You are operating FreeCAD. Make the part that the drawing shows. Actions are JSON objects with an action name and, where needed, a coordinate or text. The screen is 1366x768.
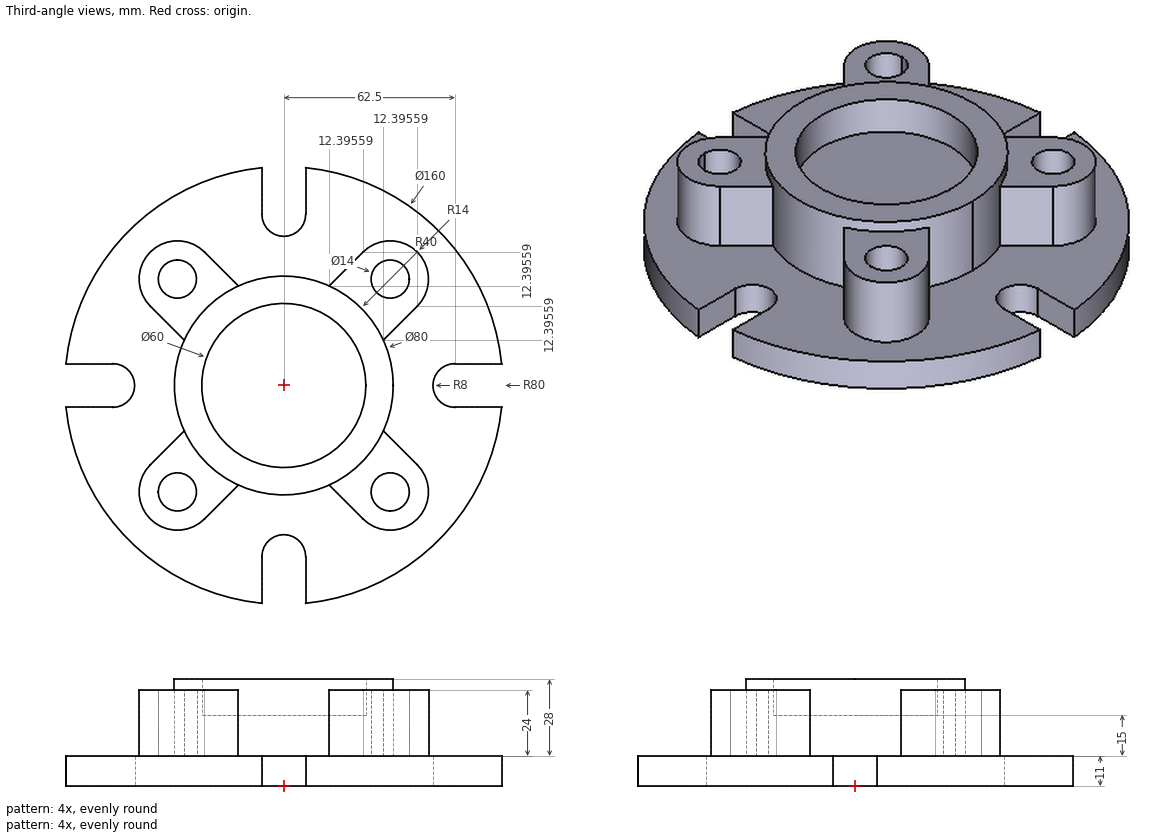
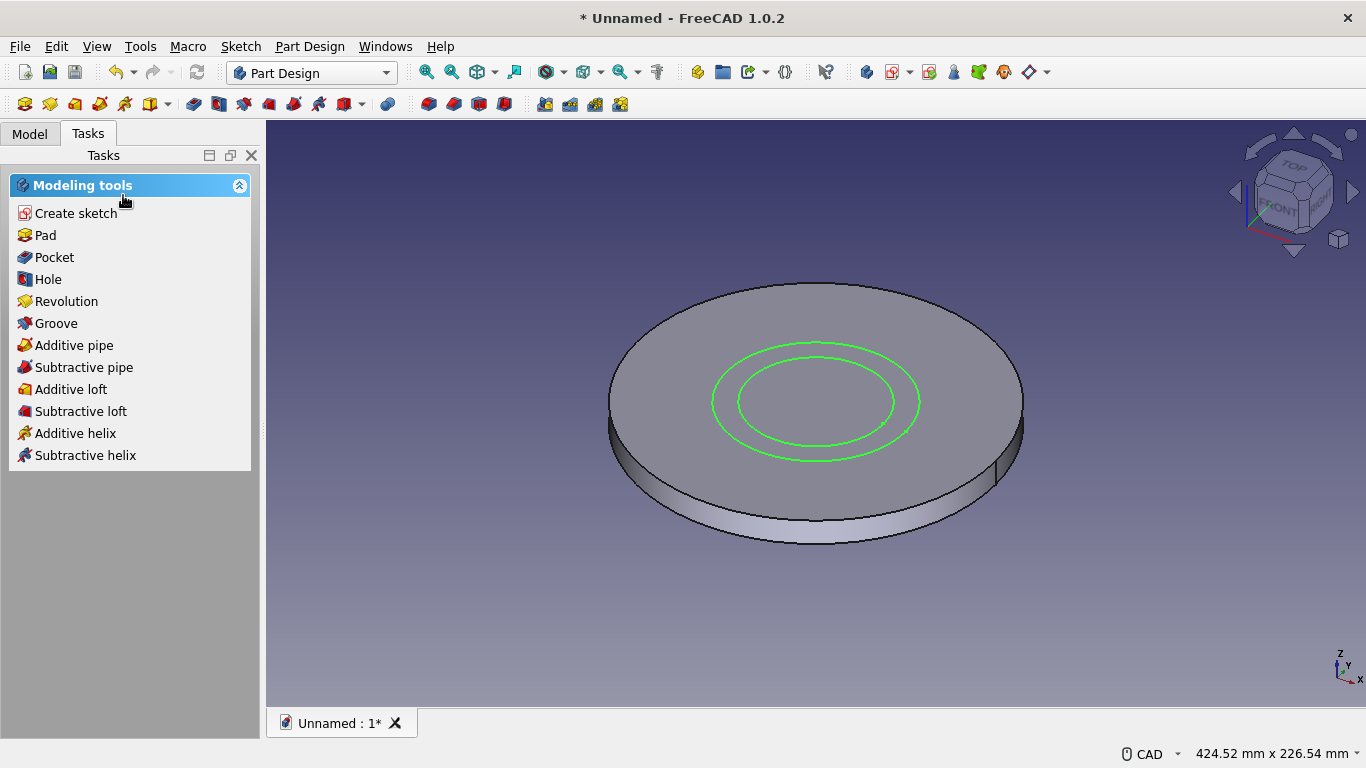
{"action": "left_click", "coordinate": [25, 104]}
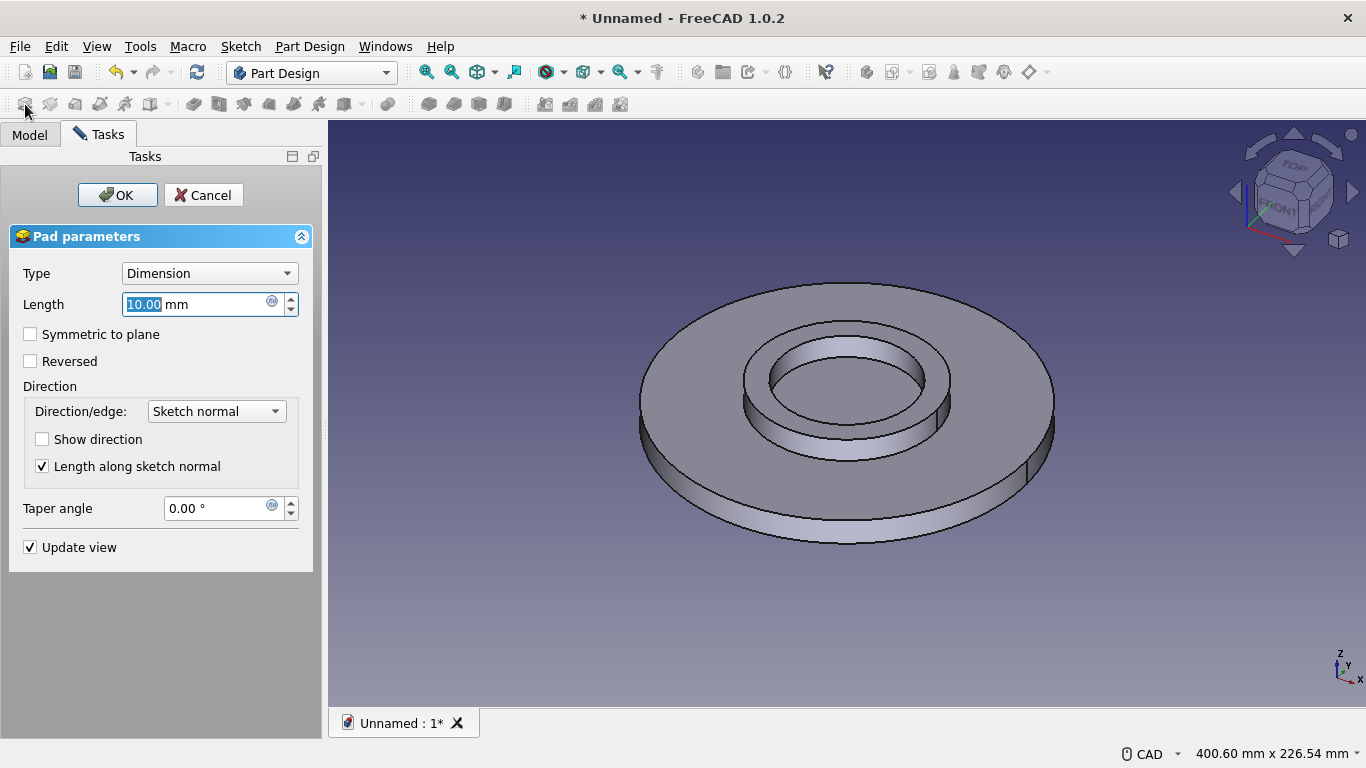
{"action": "type", "text": "28"}
{"action": "key", "text": "Tab"}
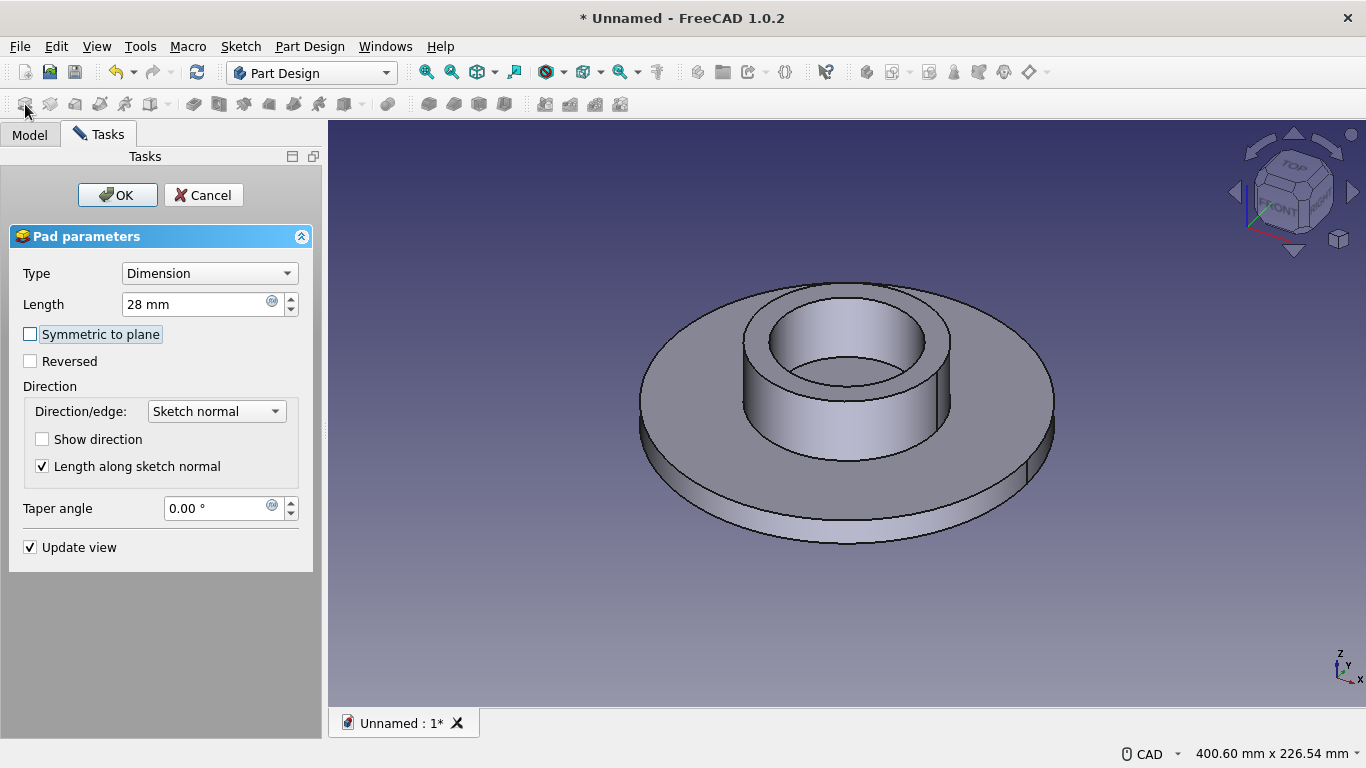
{"action": "left_click", "coordinate": [118, 195]}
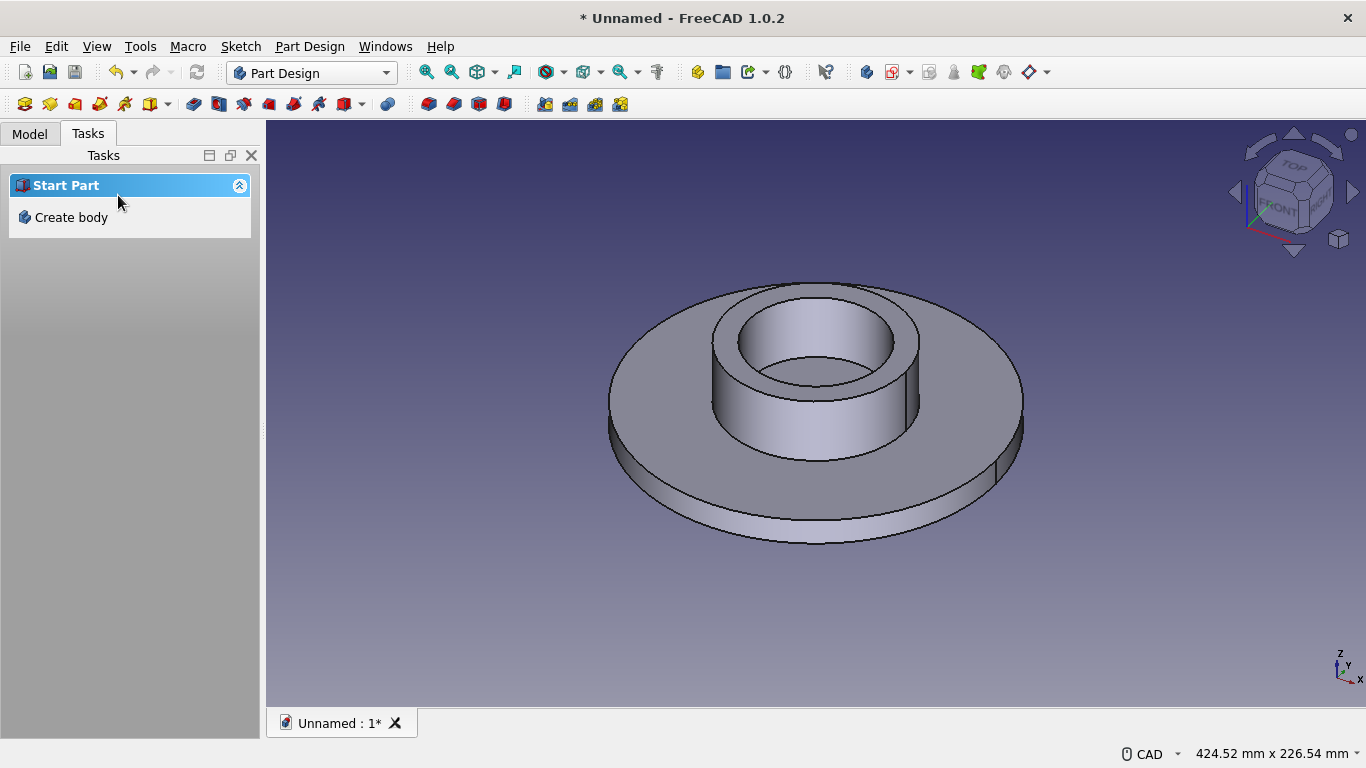
{"action": "left_click", "coordinate": [859, 493]}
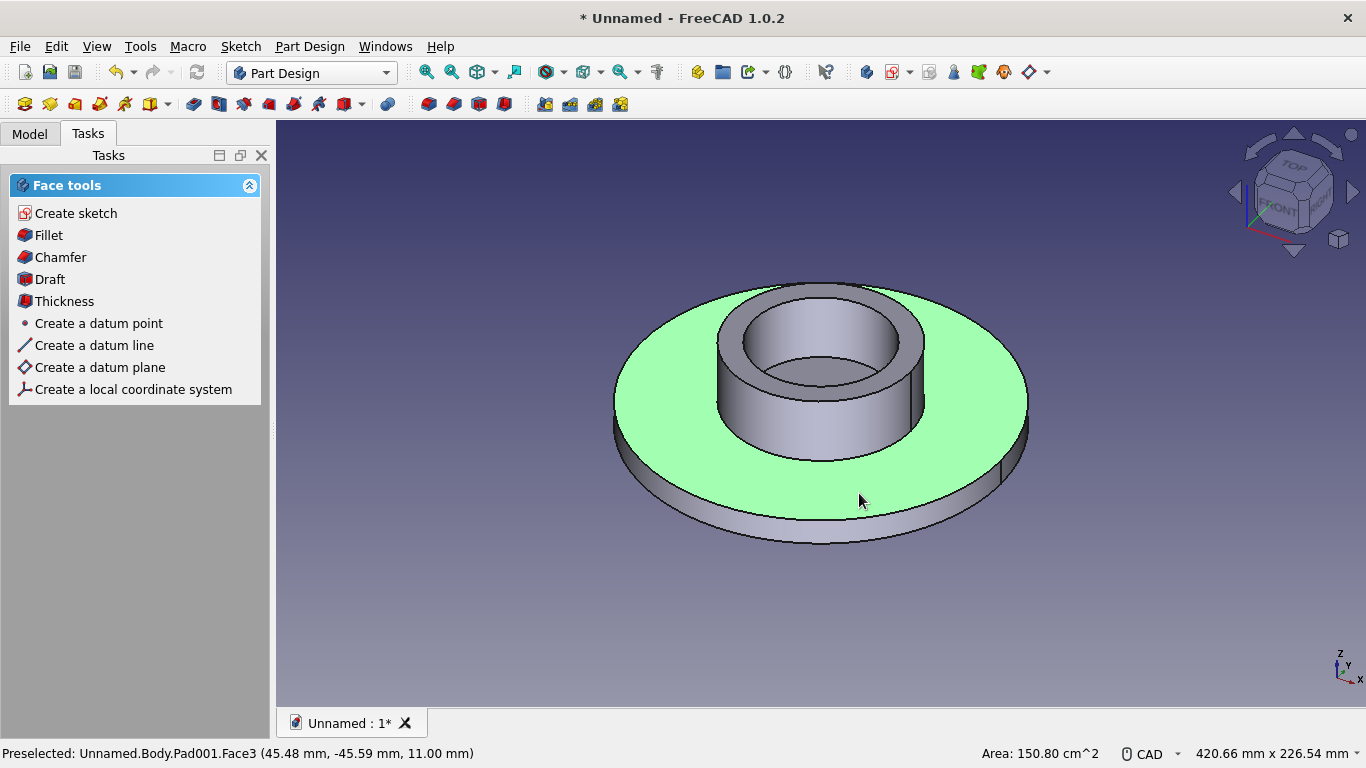
{"action": "left_click", "coordinate": [892, 72]}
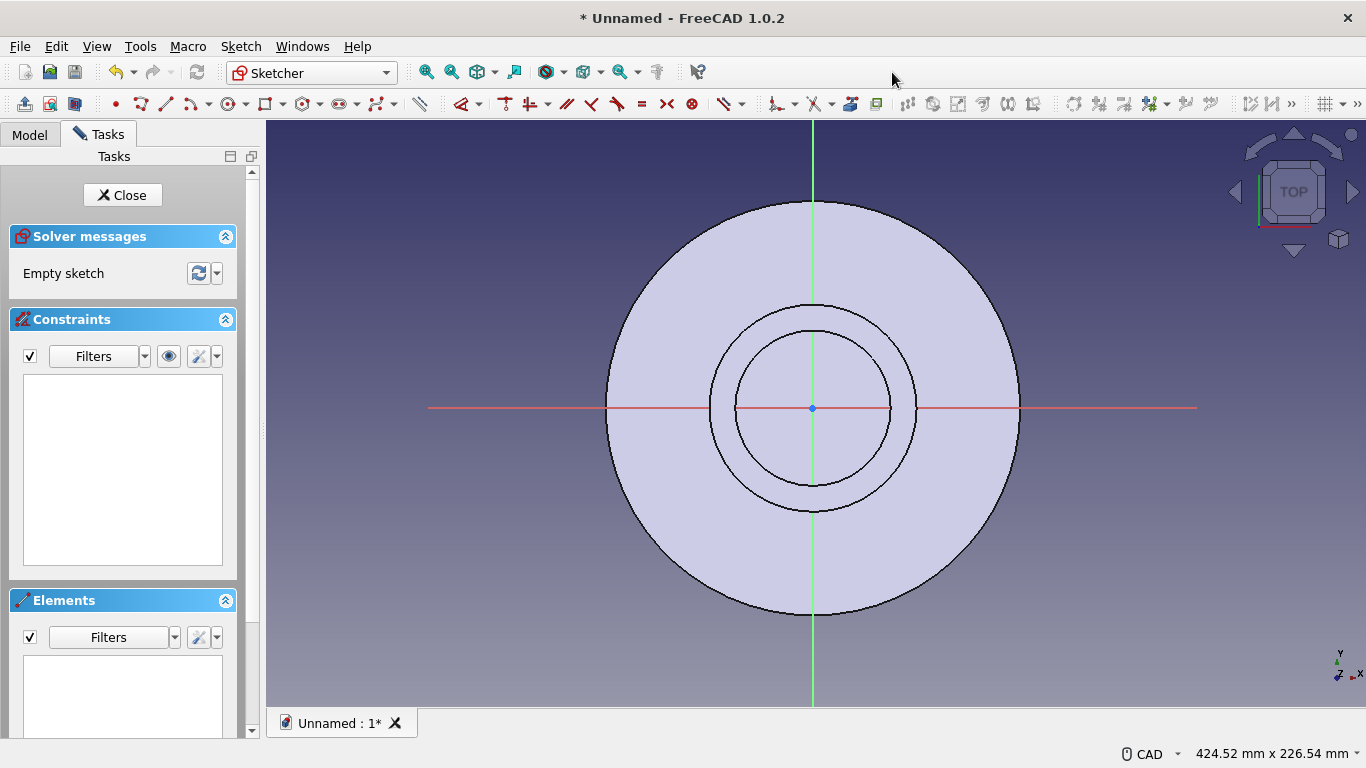
{"action": "left_click", "coordinate": [75, 104]}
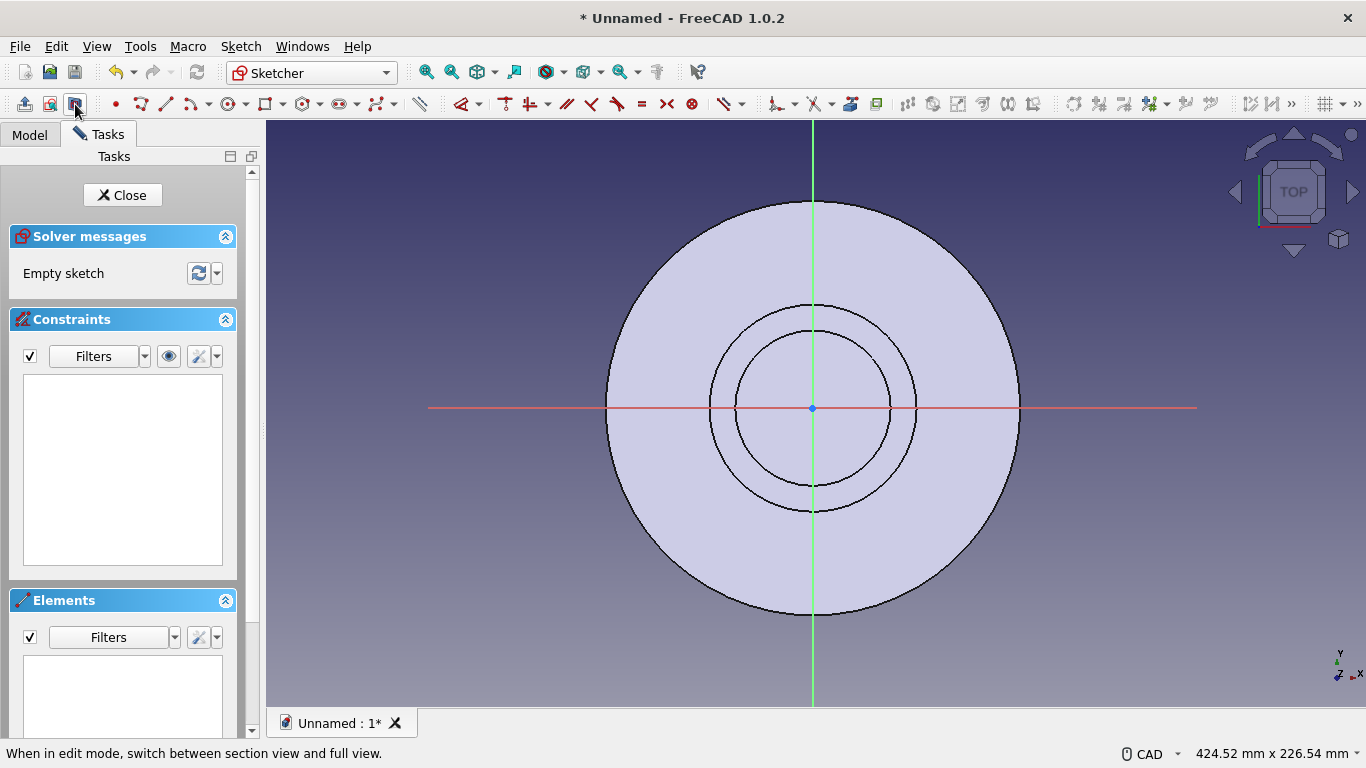
{"action": "scroll", "coordinate": [866, 404], "scroll_direction": "up", "scroll_amount": 4}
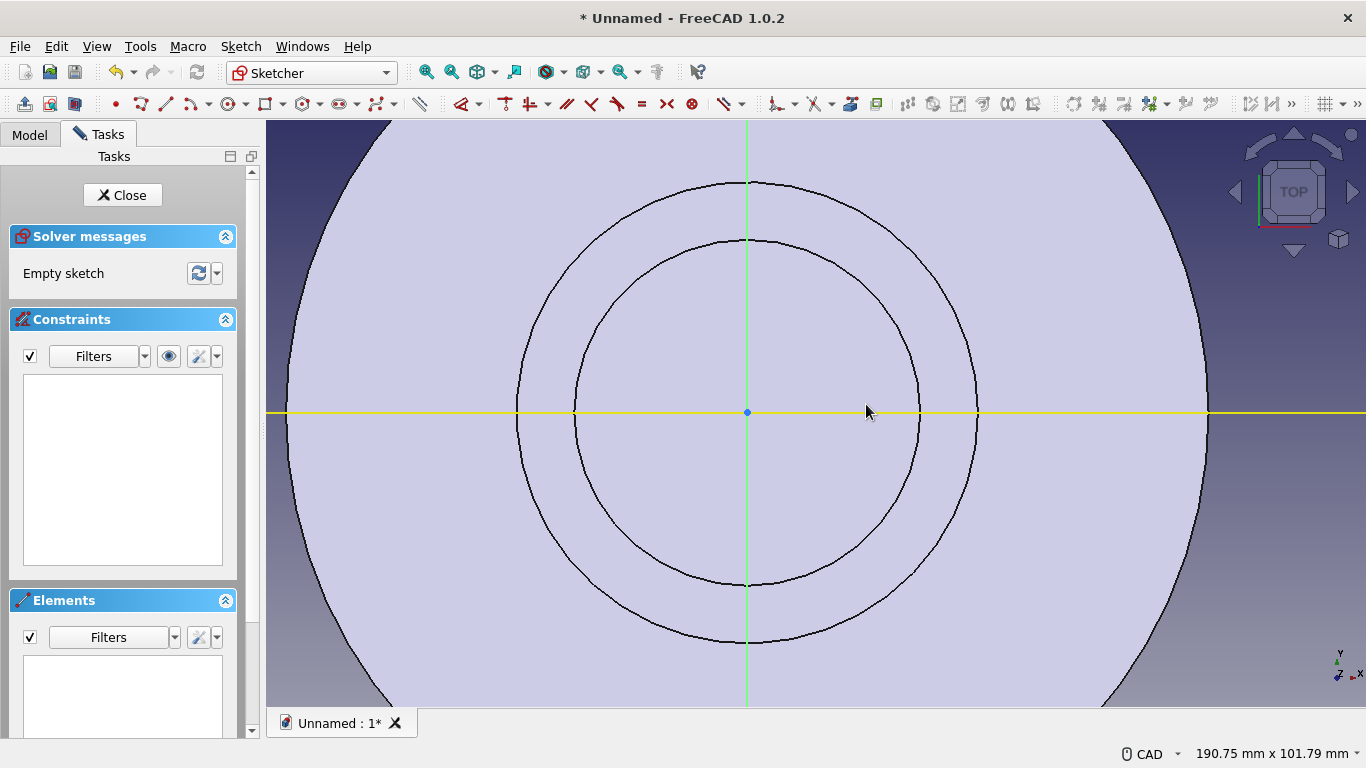
{"action": "key", "text": "g c"}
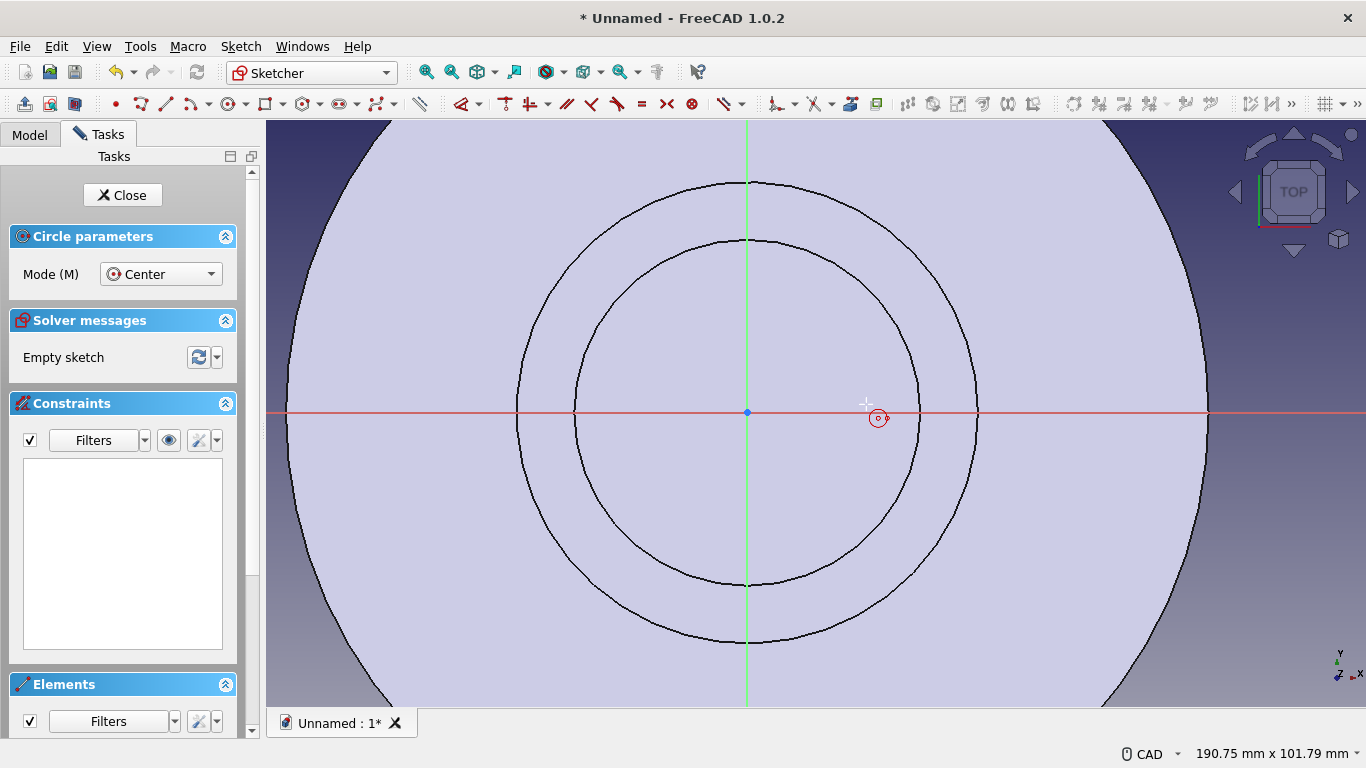
{"action": "left_click", "coordinate": [747, 413]}
{"action": "left_click", "coordinate": [870, 290]}
{"action": "key", "text": "Escape"}